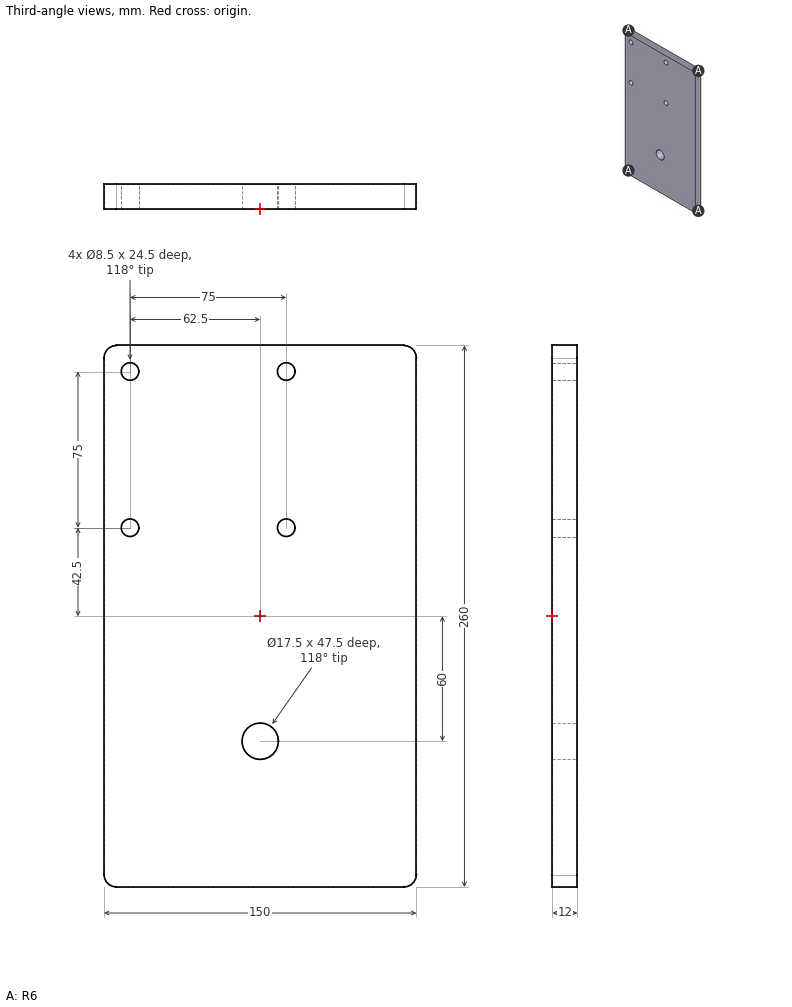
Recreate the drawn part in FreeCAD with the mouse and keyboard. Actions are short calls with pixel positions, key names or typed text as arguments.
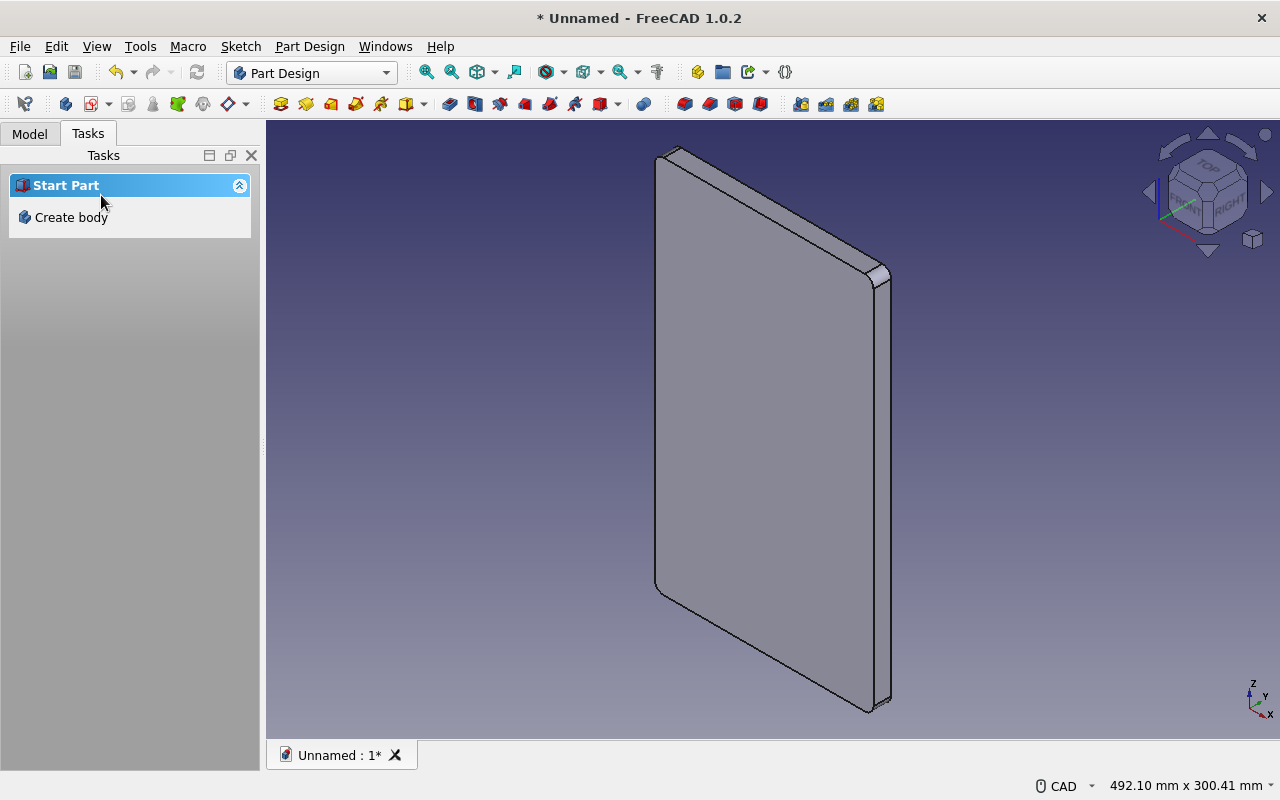
click(764, 371)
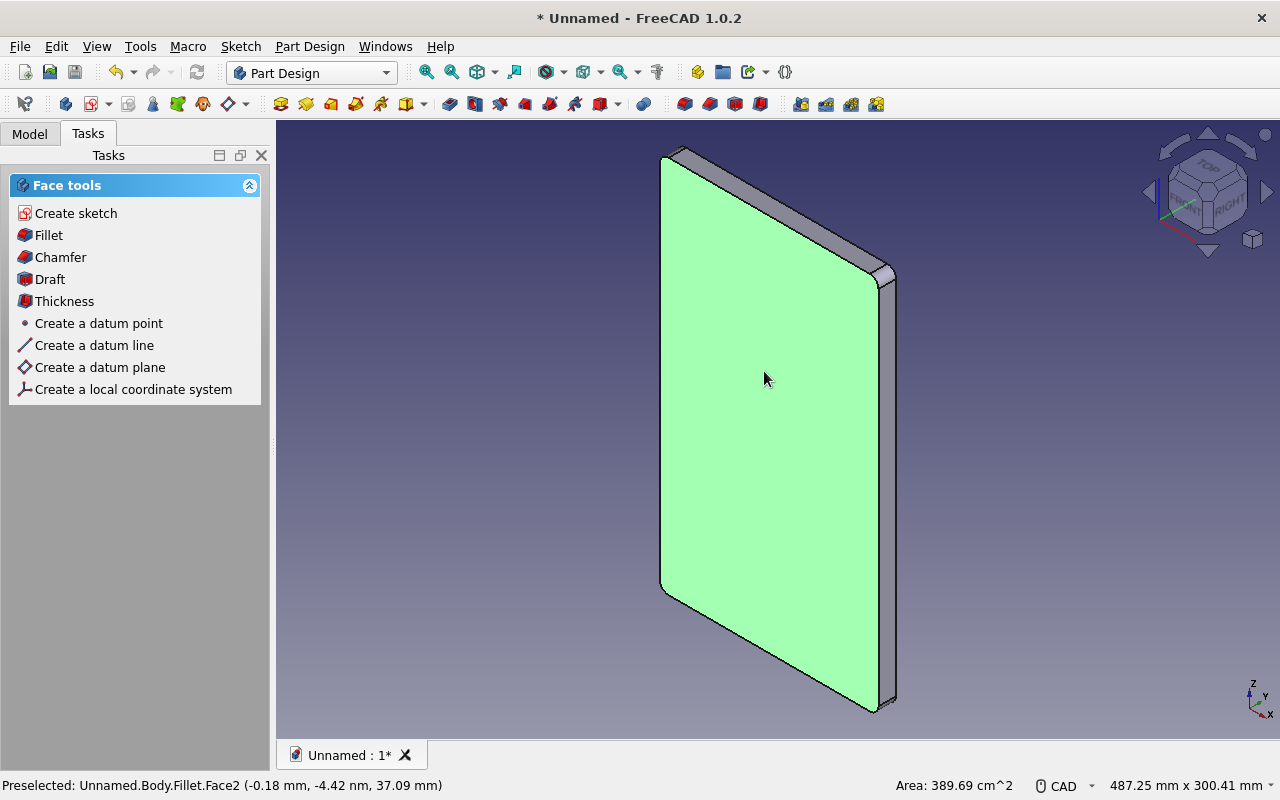
click(90, 104)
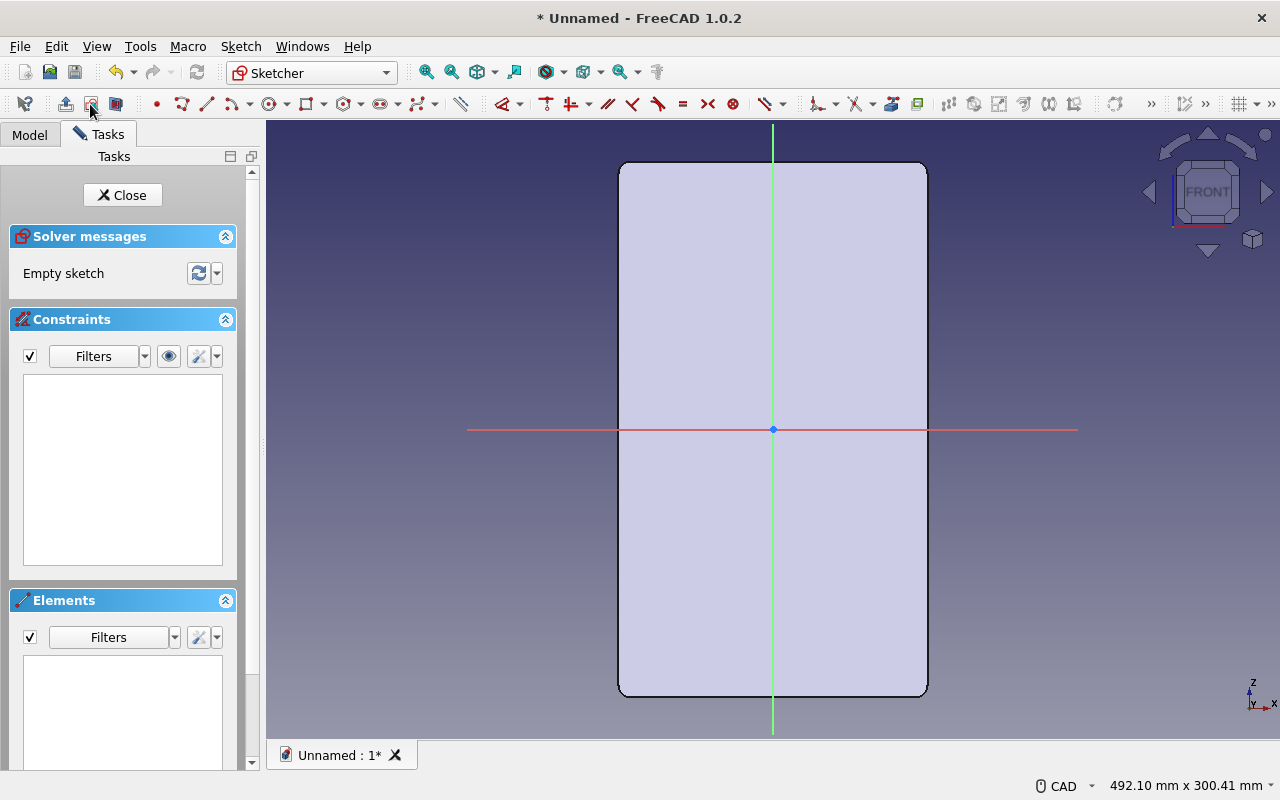
scroll(780, 565, up, 12)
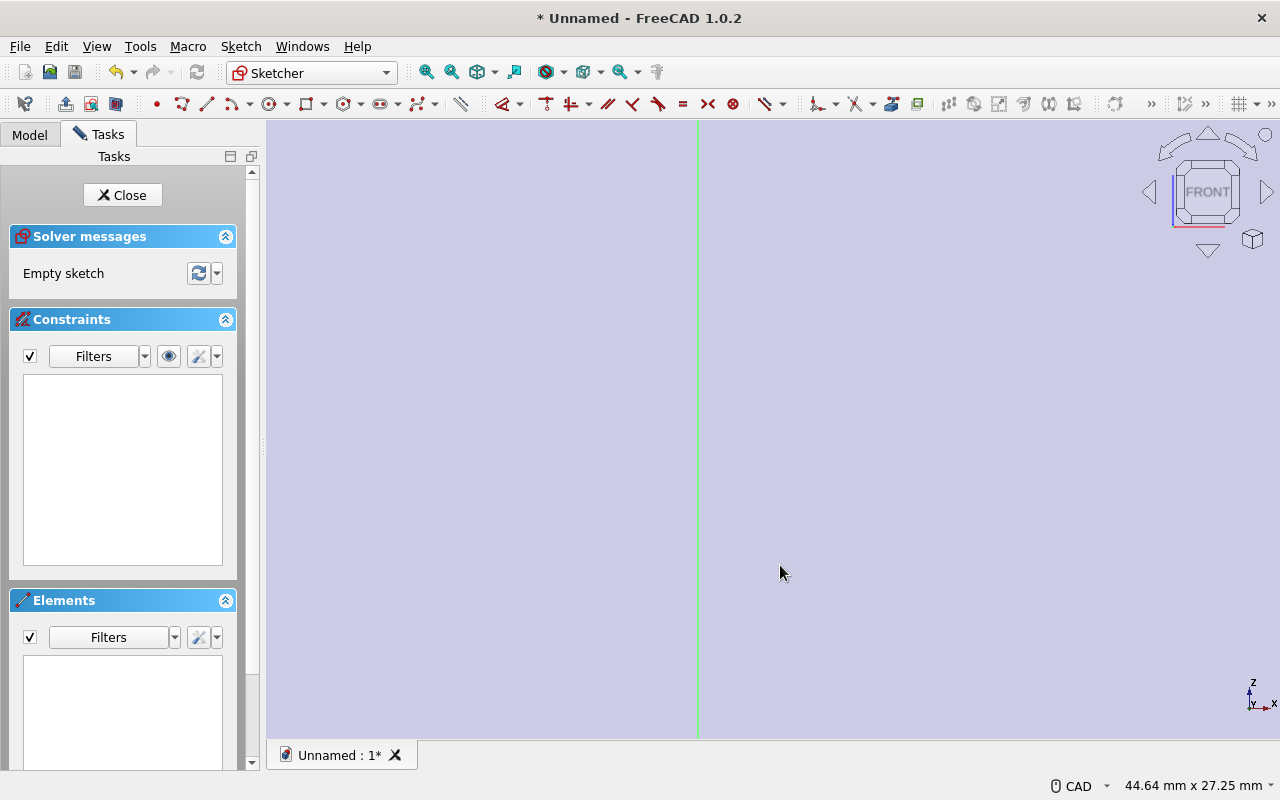
click(268, 104)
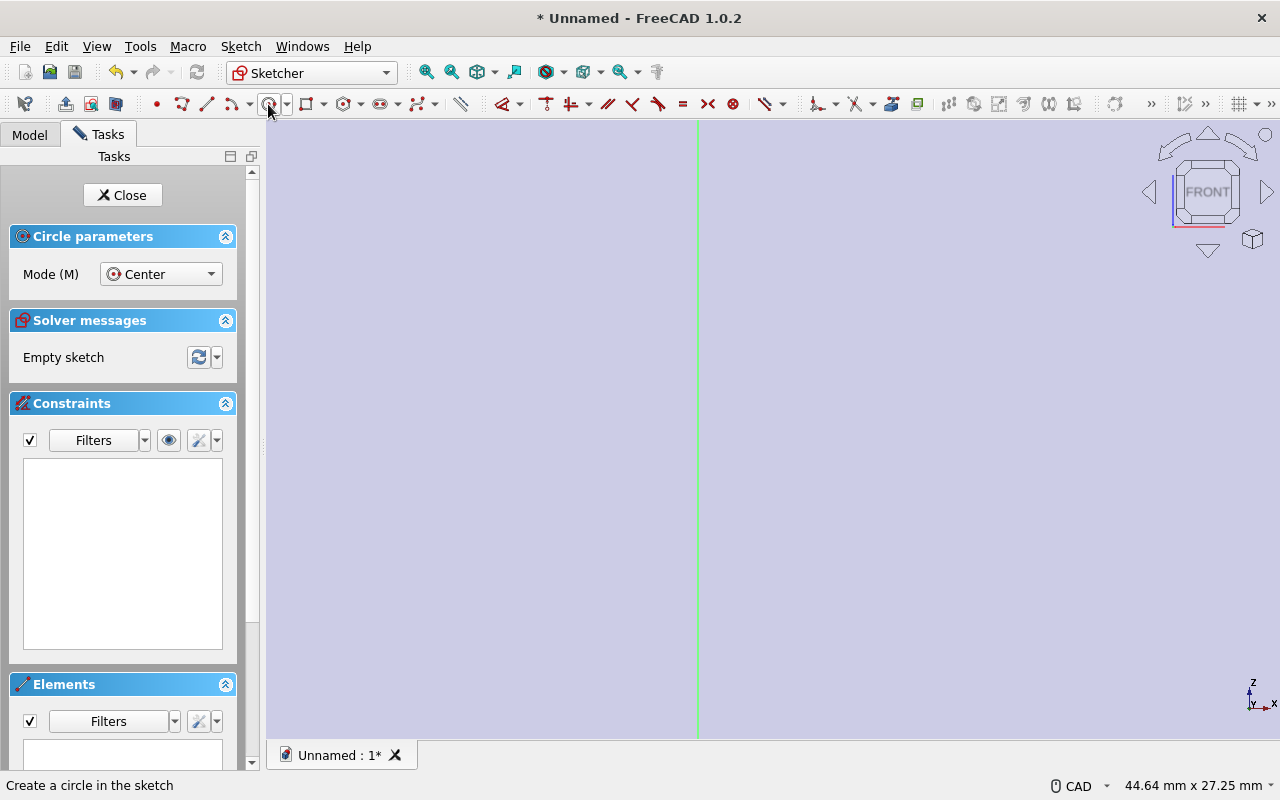
click(698, 427)
move(838, 286)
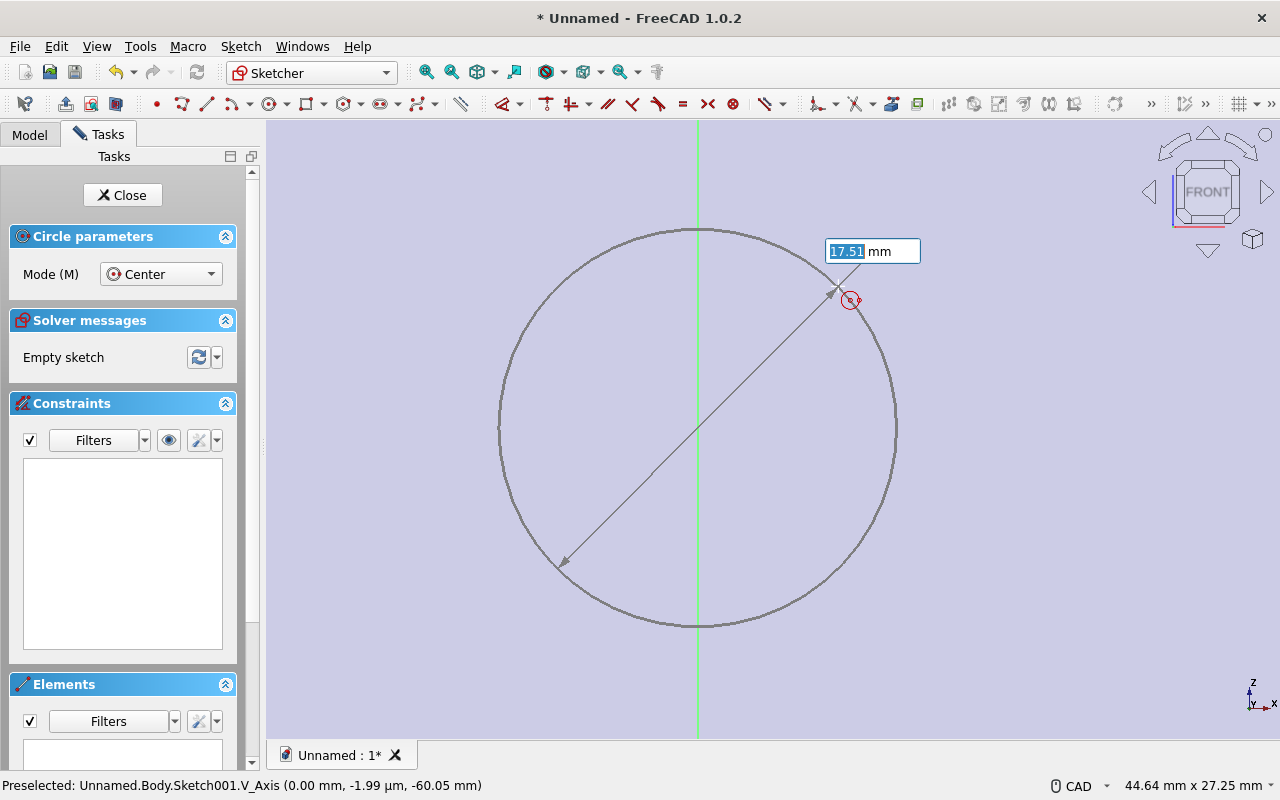
text(17.5)
key(Return)
key(Escape)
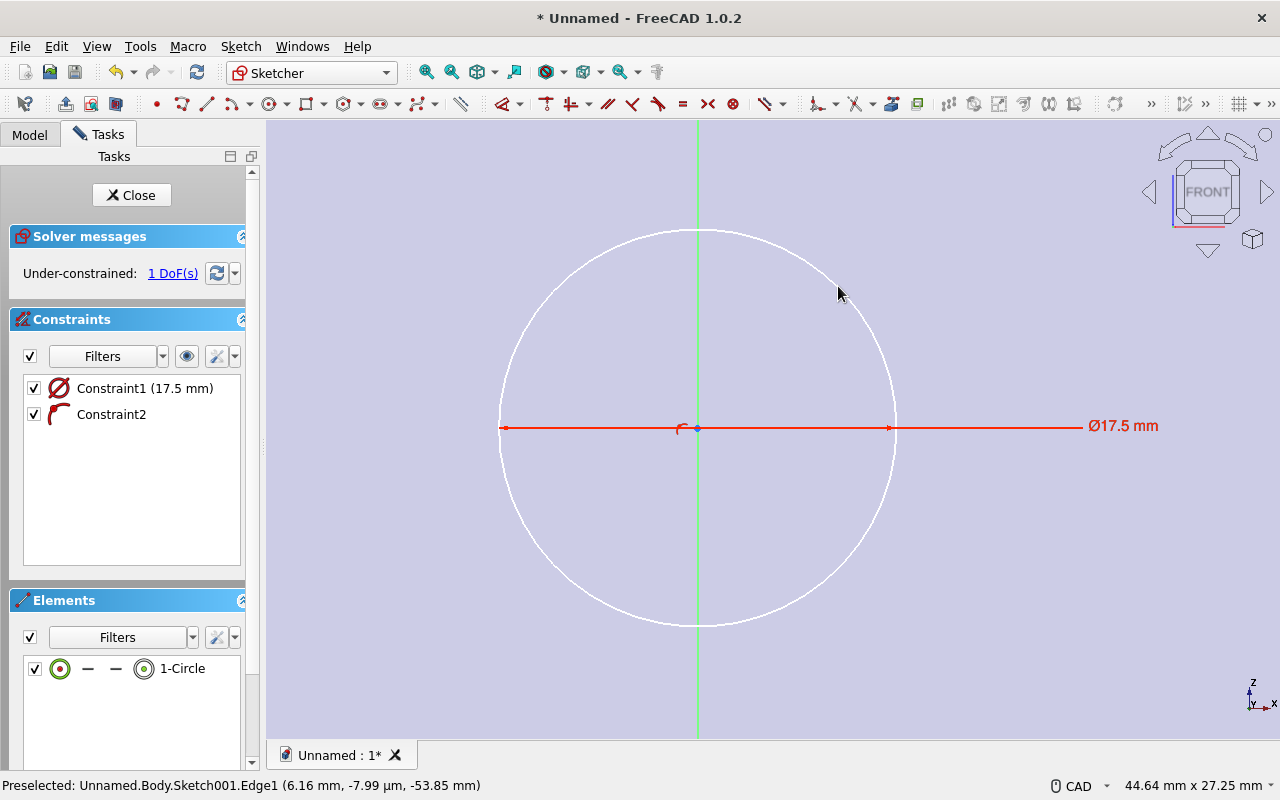
key(d)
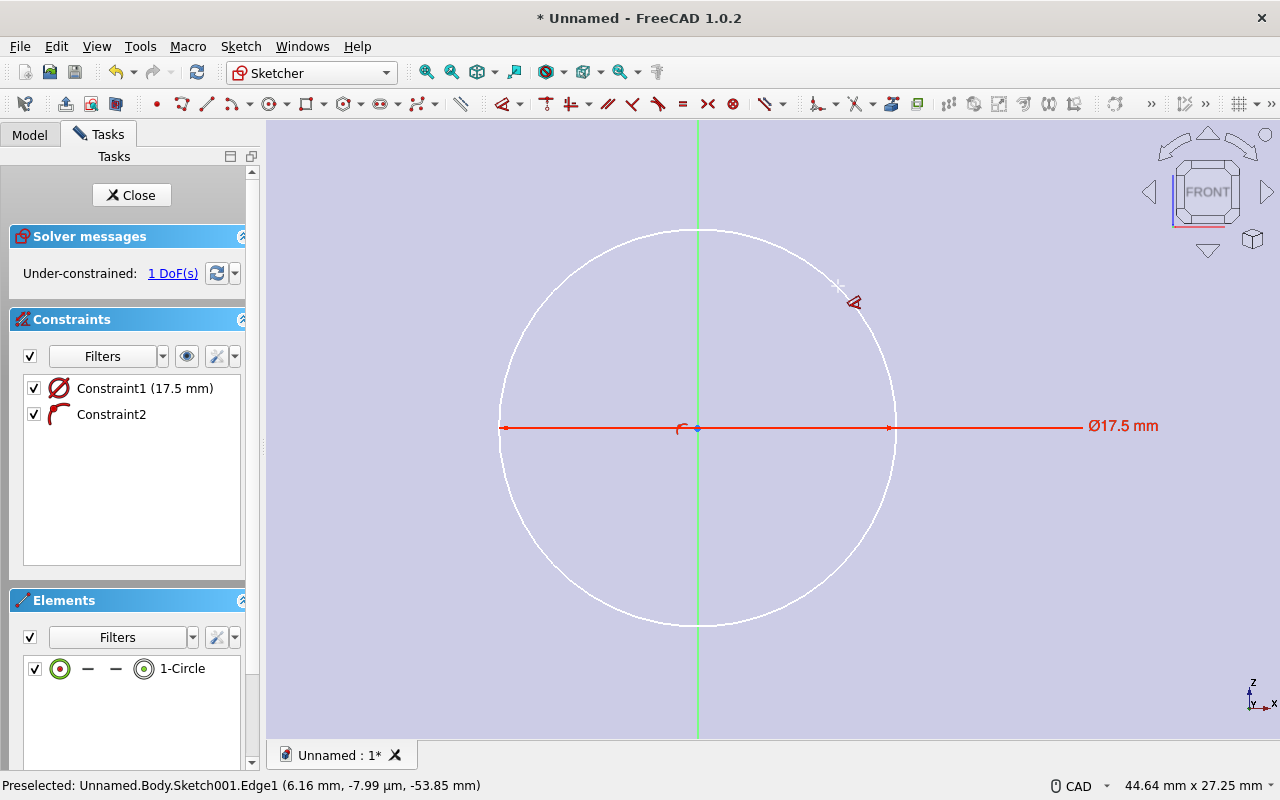
click(698, 428)
click(732, 288)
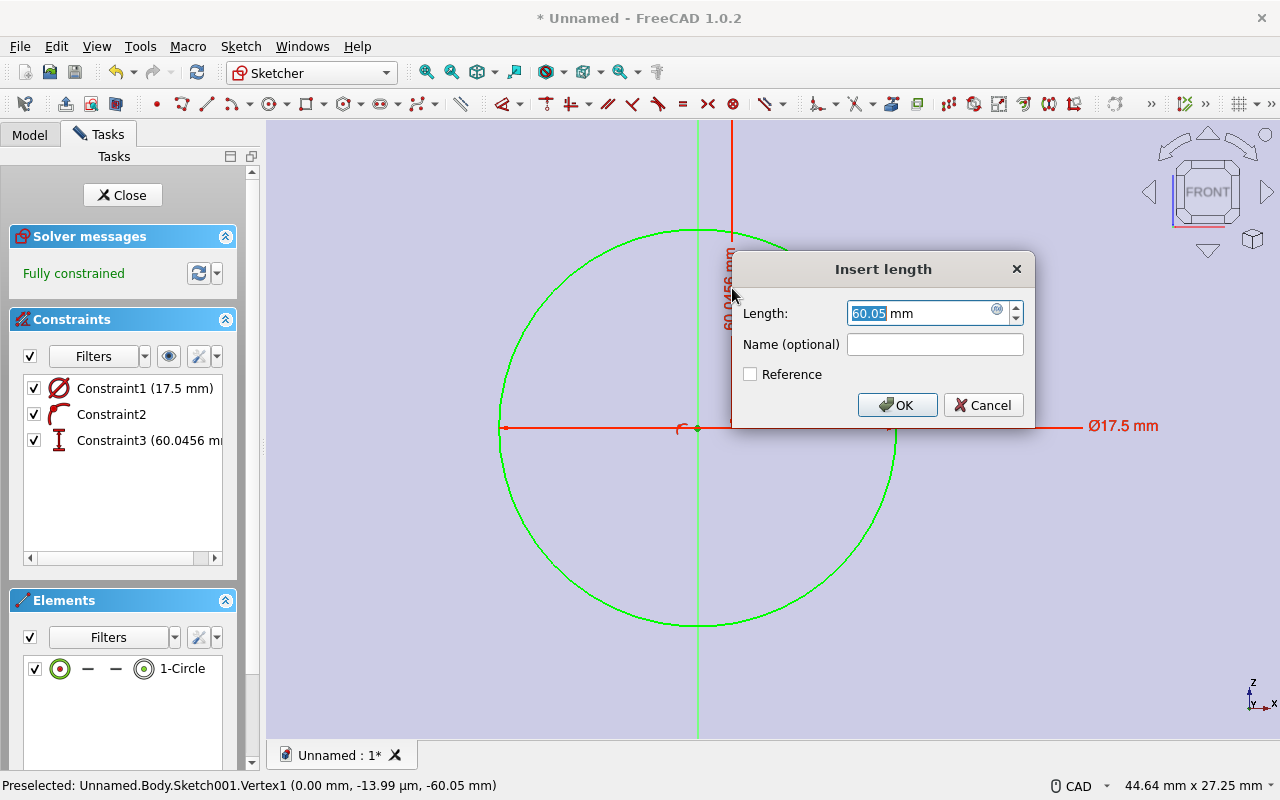
text(60)
key(Return)
key(Escape)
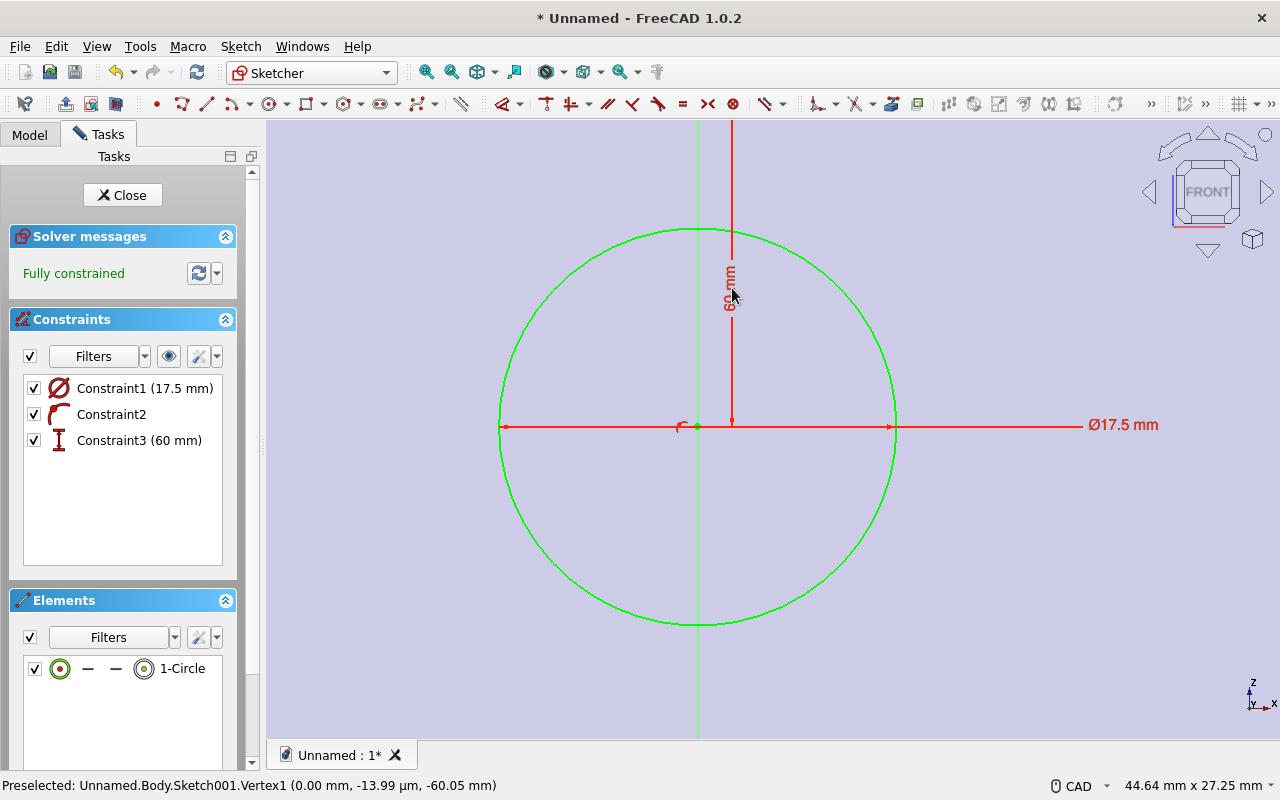
click(123, 195)